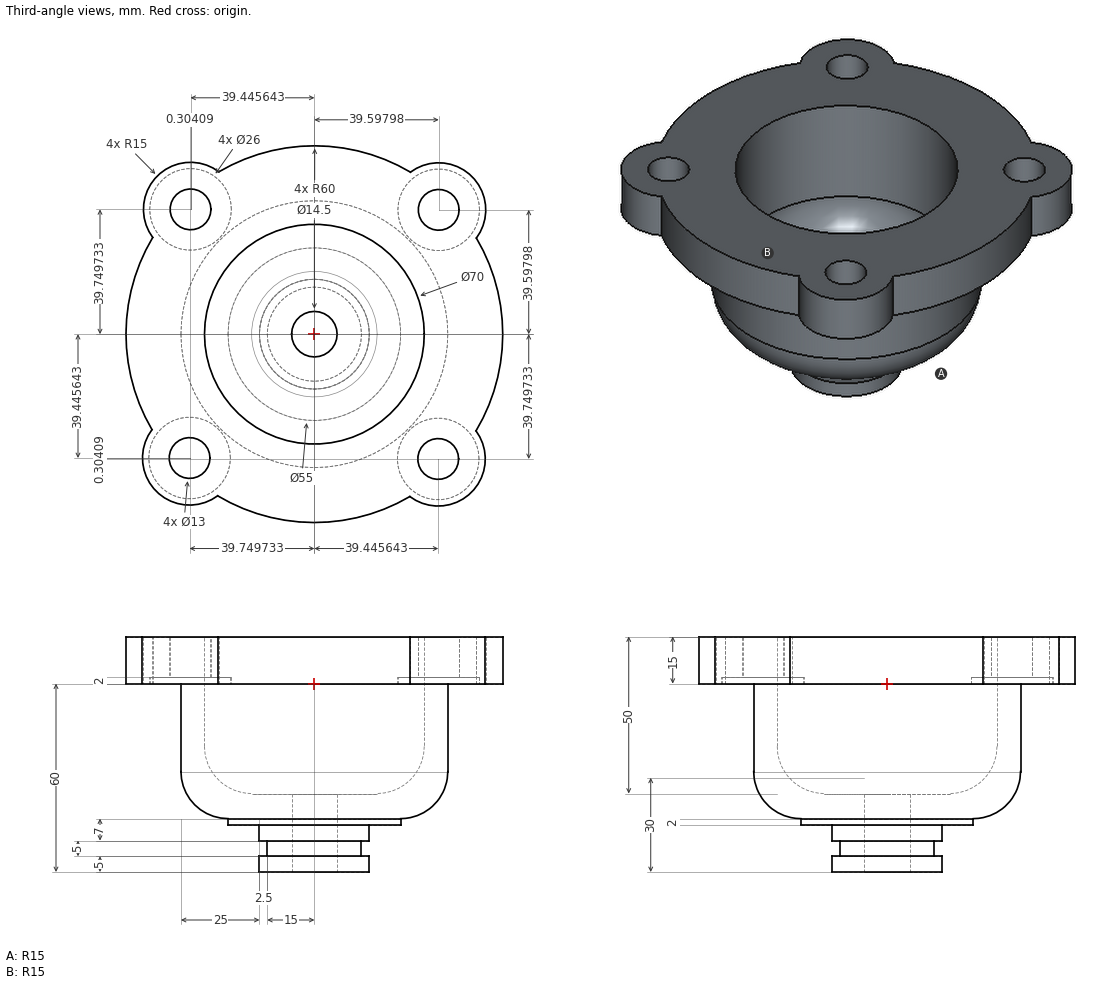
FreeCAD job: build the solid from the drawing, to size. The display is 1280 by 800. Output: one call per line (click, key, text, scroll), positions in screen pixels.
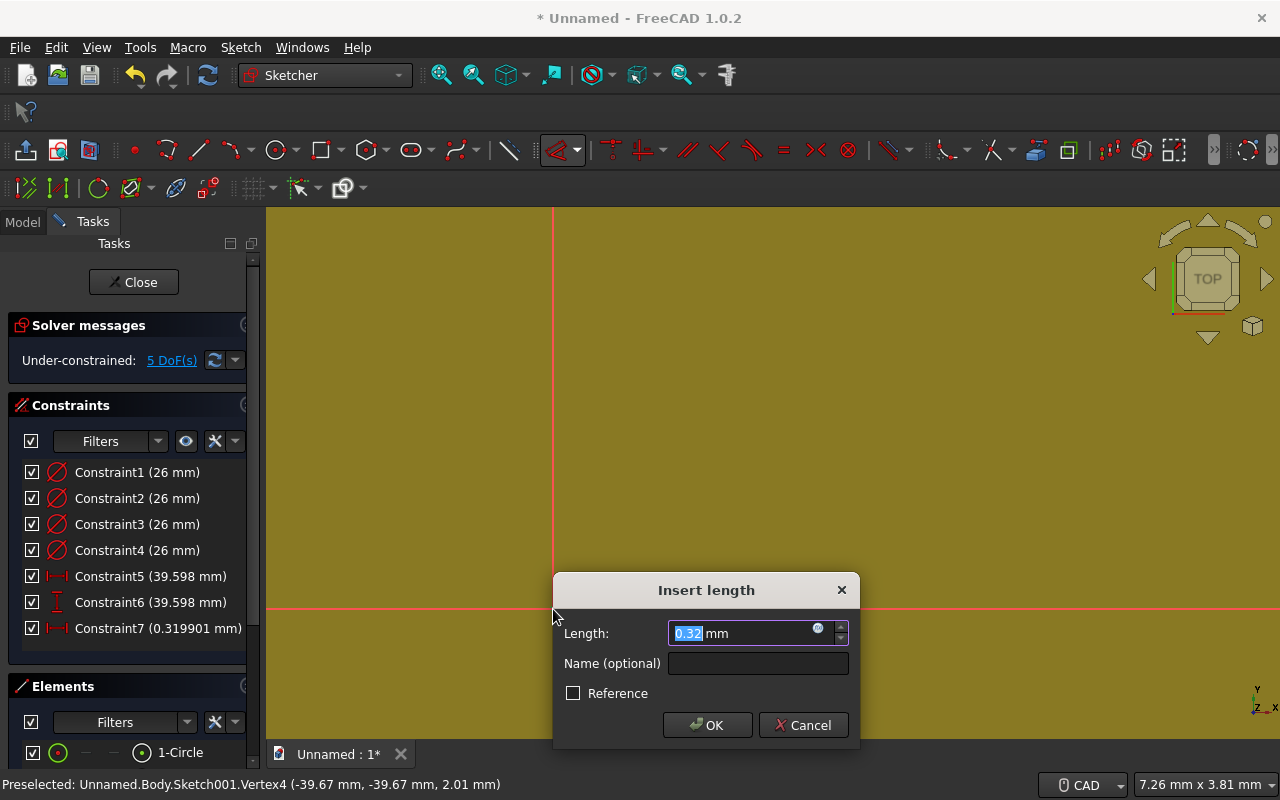
text(0.30409)
key(Return)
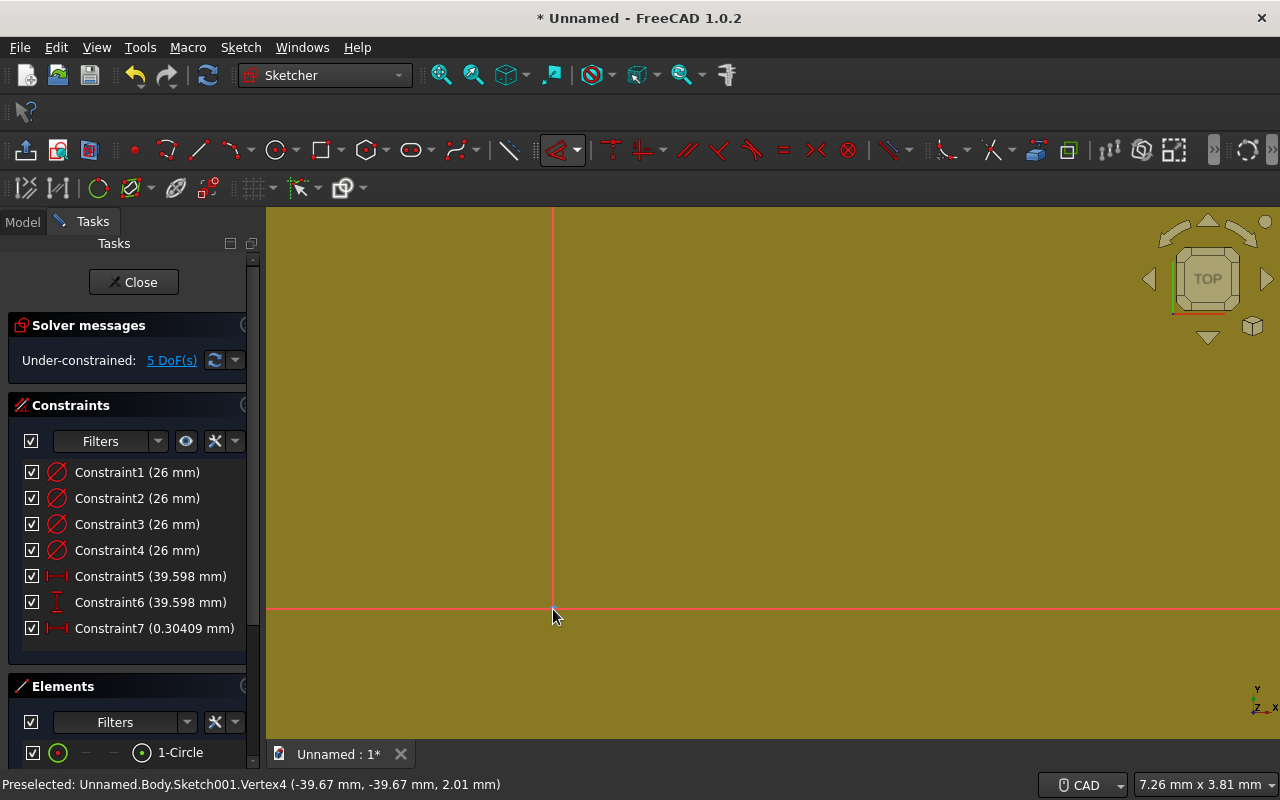
scroll(553, 625, down, 18)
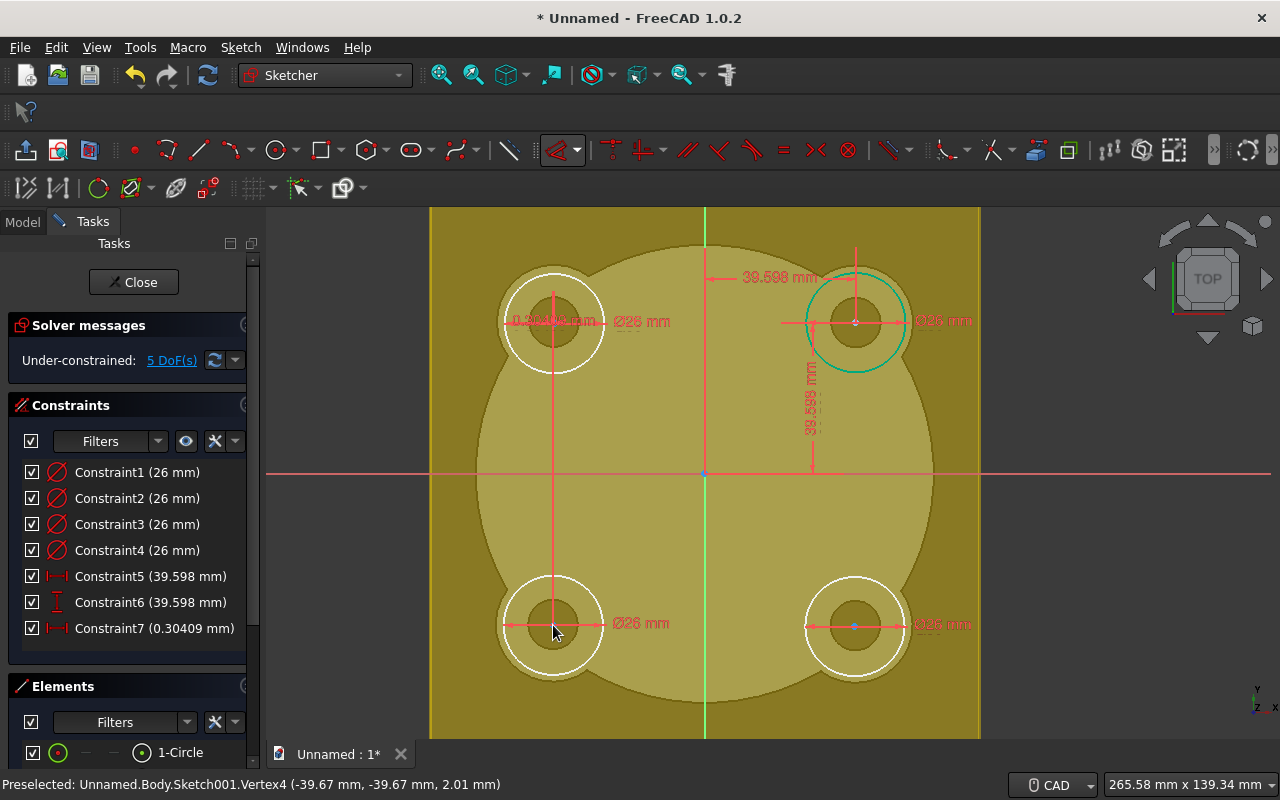
scroll(855, 627, up, 18)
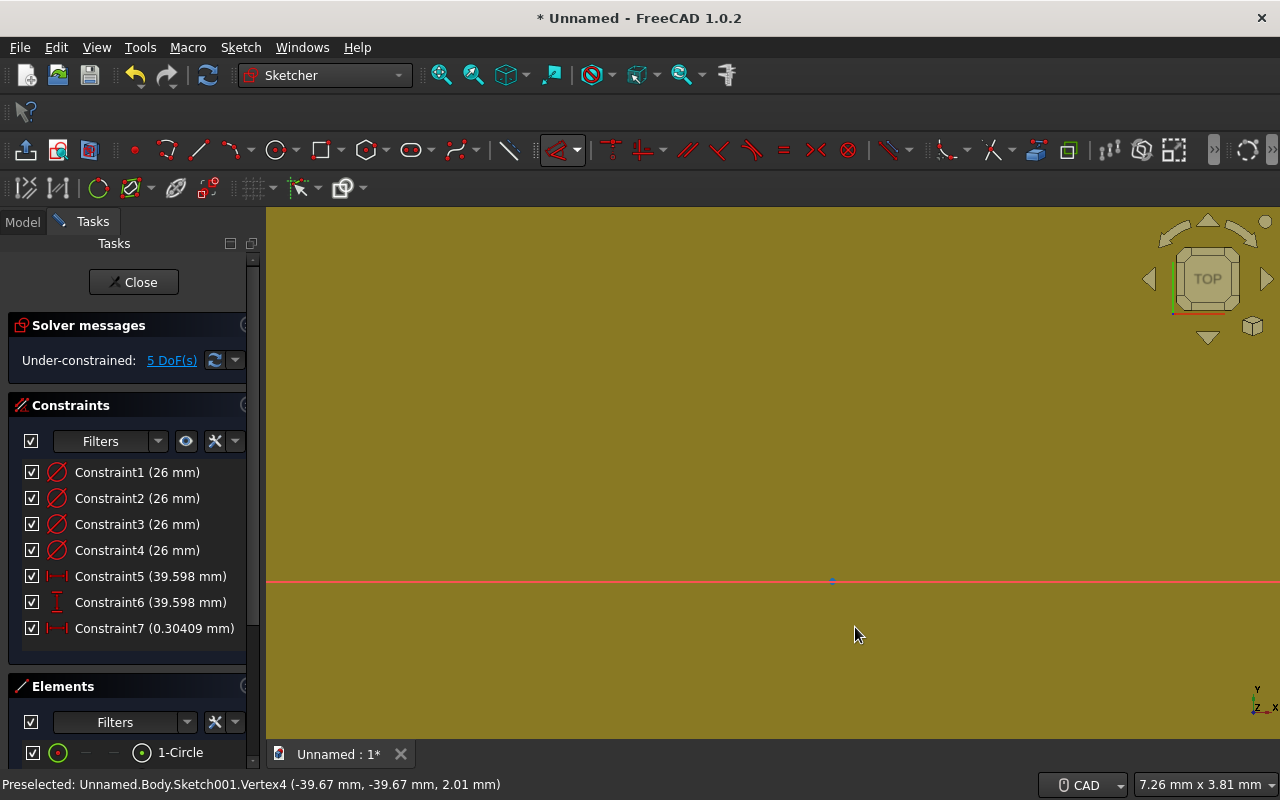
click(833, 582)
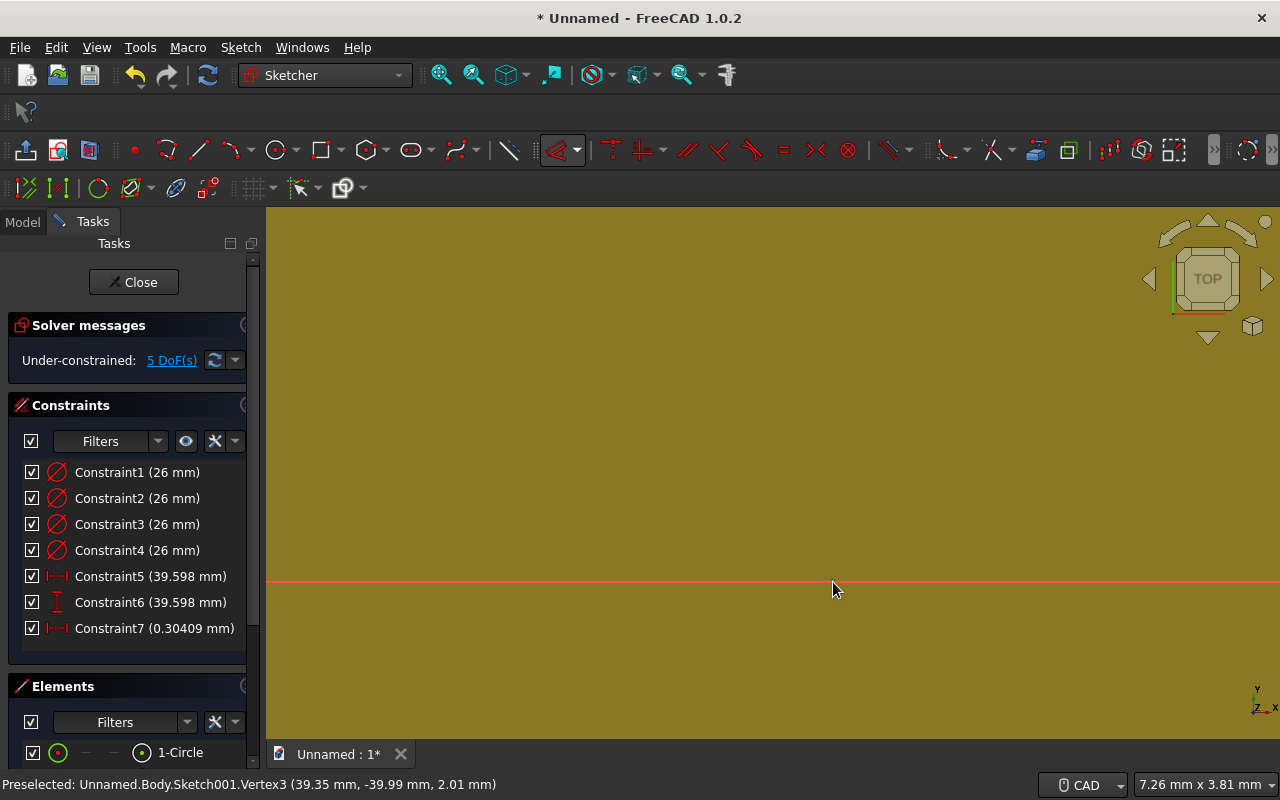
scroll(856, 627, down, 18)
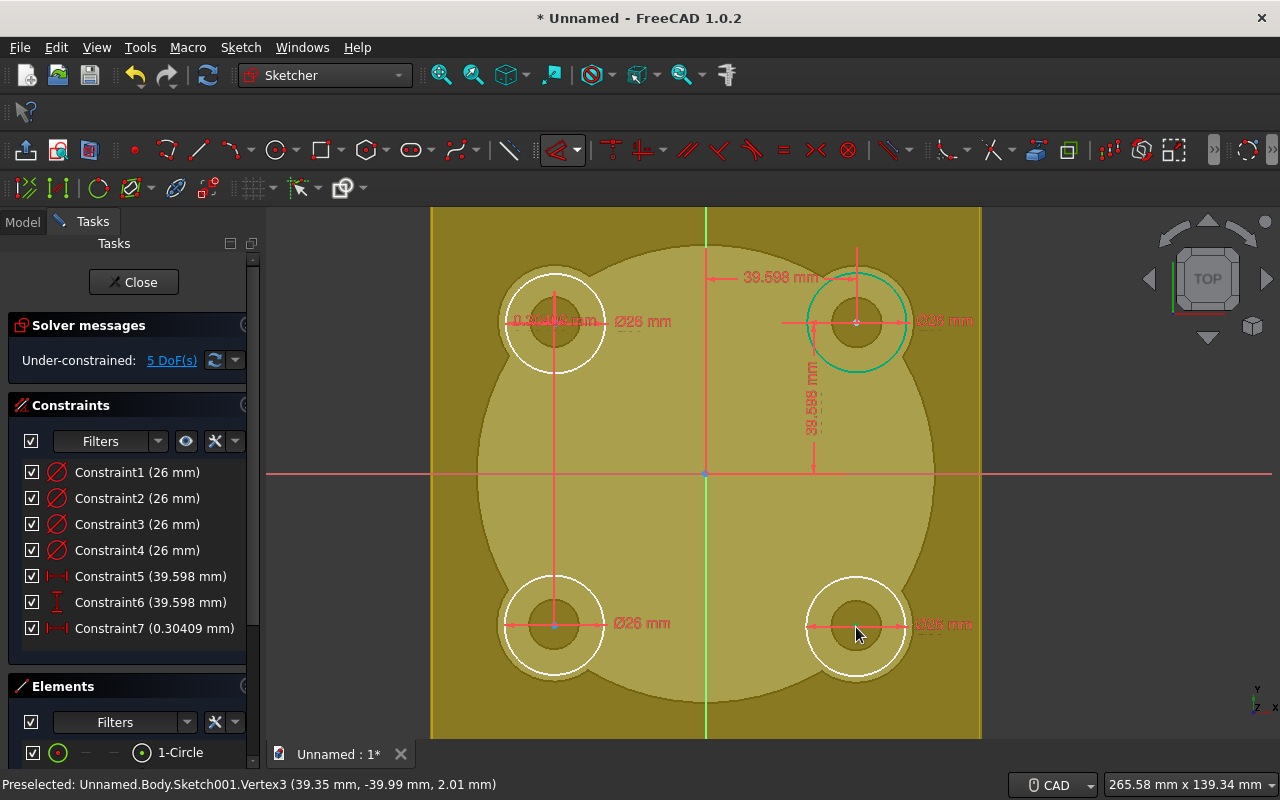
scroll(554, 625, up, 18)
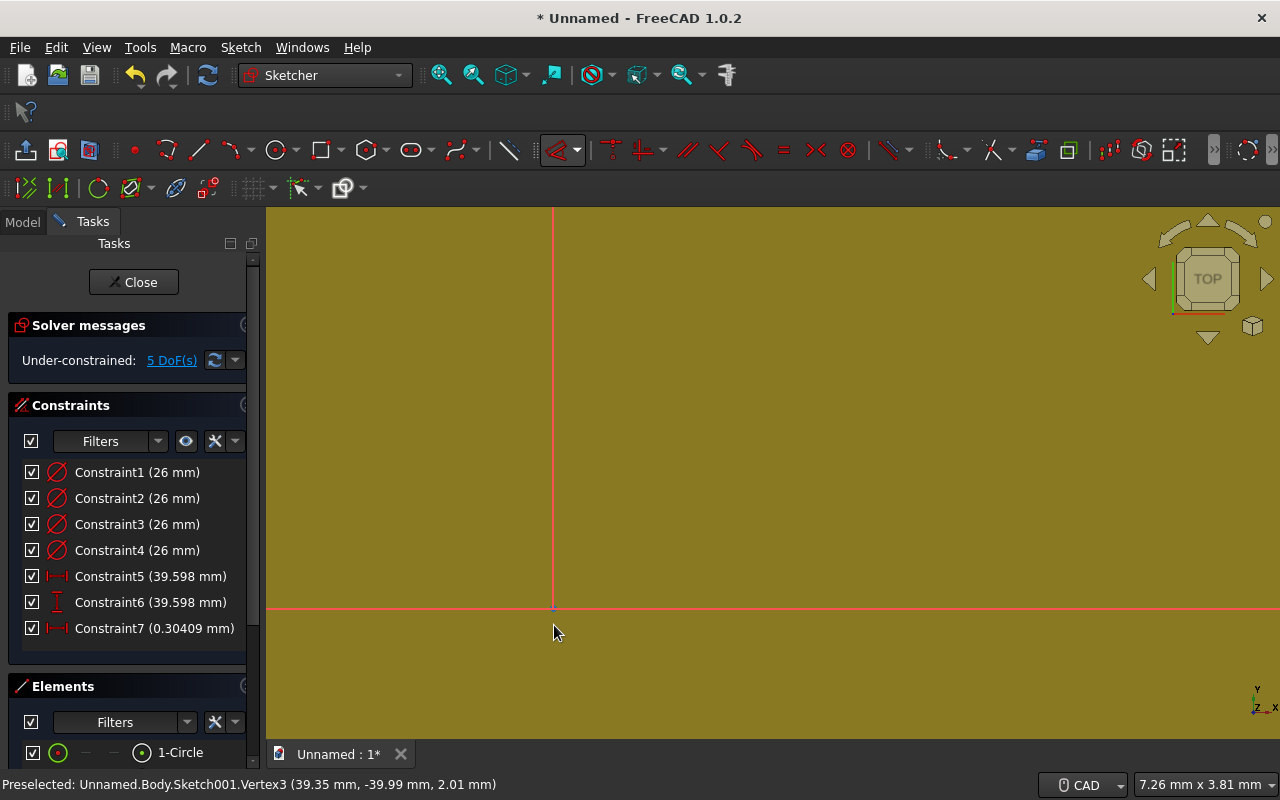
click(553, 609)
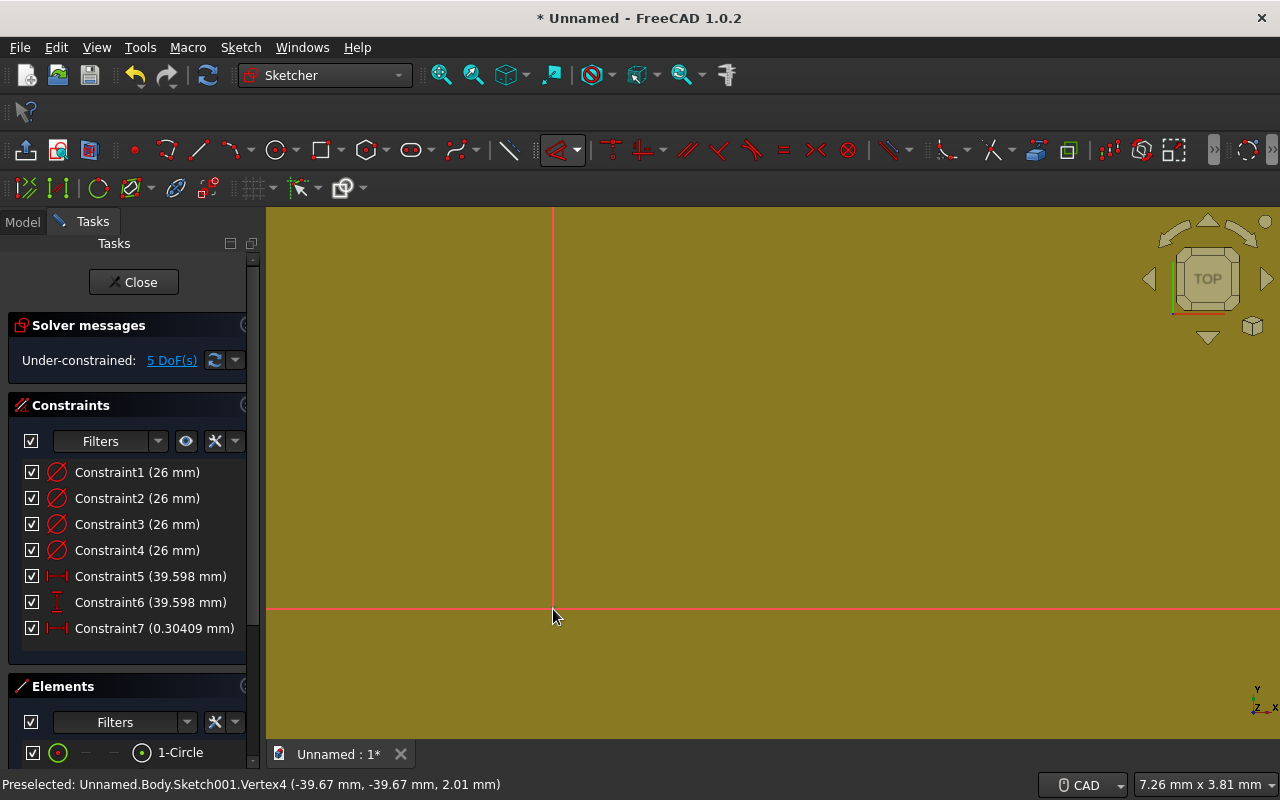
key(i)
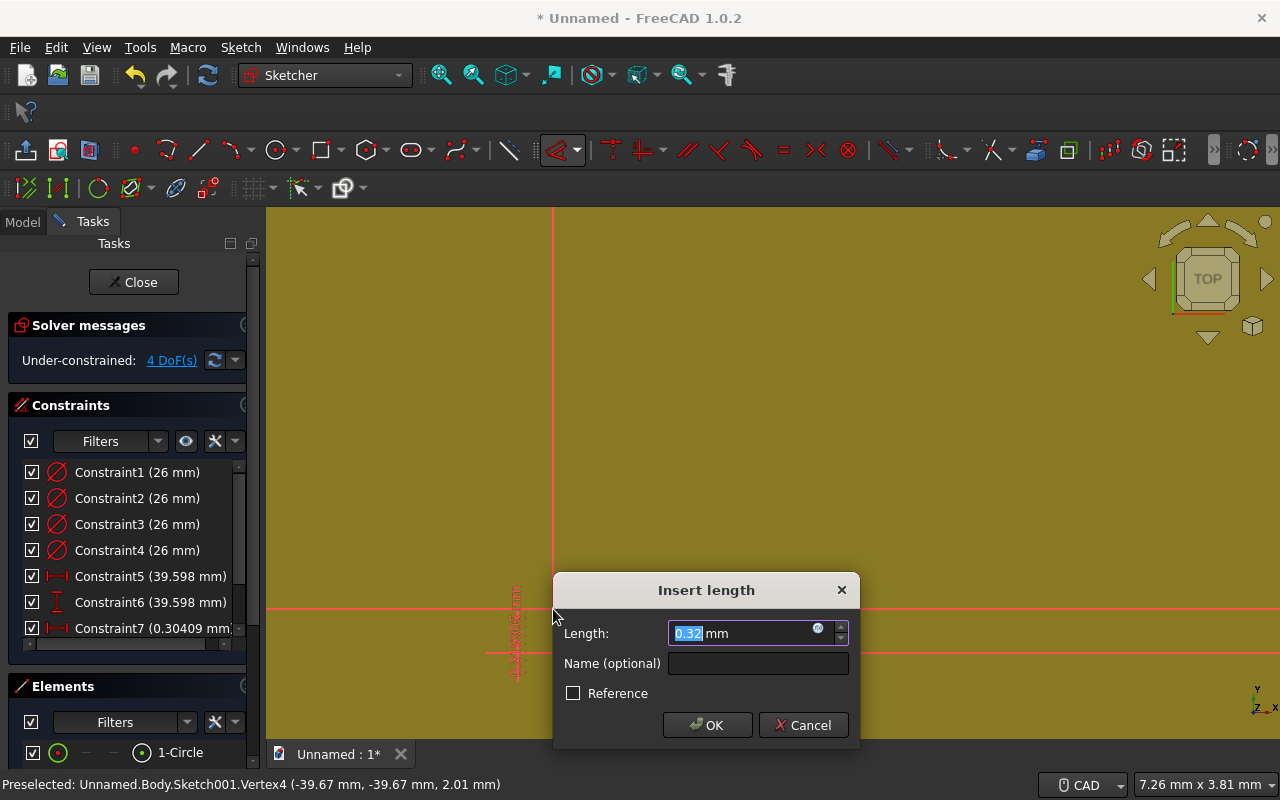
text(0.30409)
key(Return)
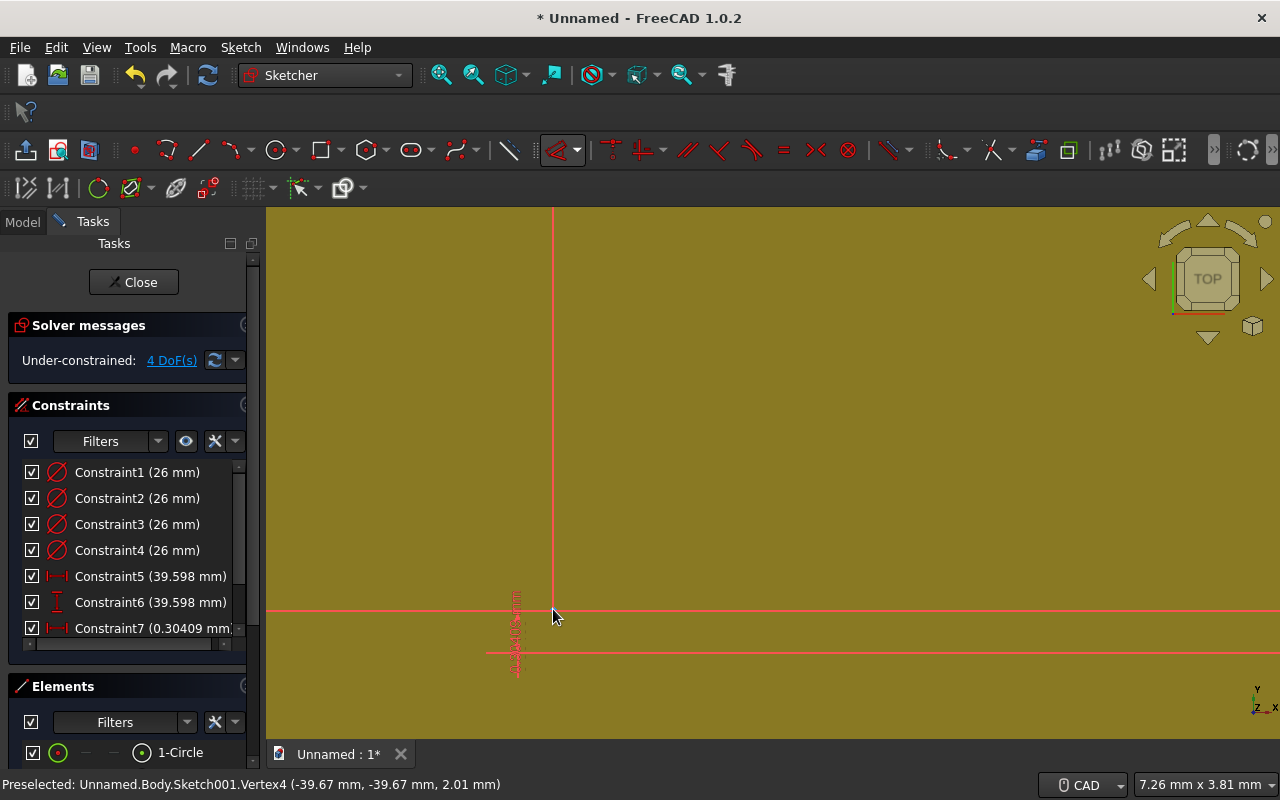
scroll(553, 625, down, 18)